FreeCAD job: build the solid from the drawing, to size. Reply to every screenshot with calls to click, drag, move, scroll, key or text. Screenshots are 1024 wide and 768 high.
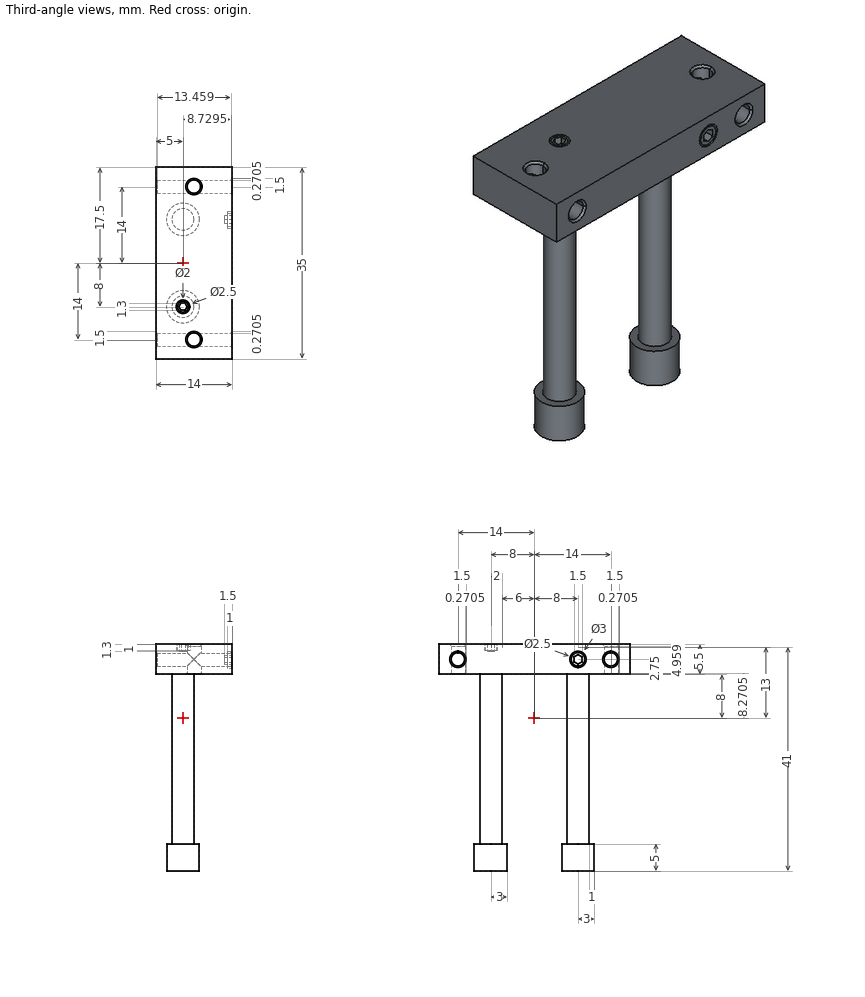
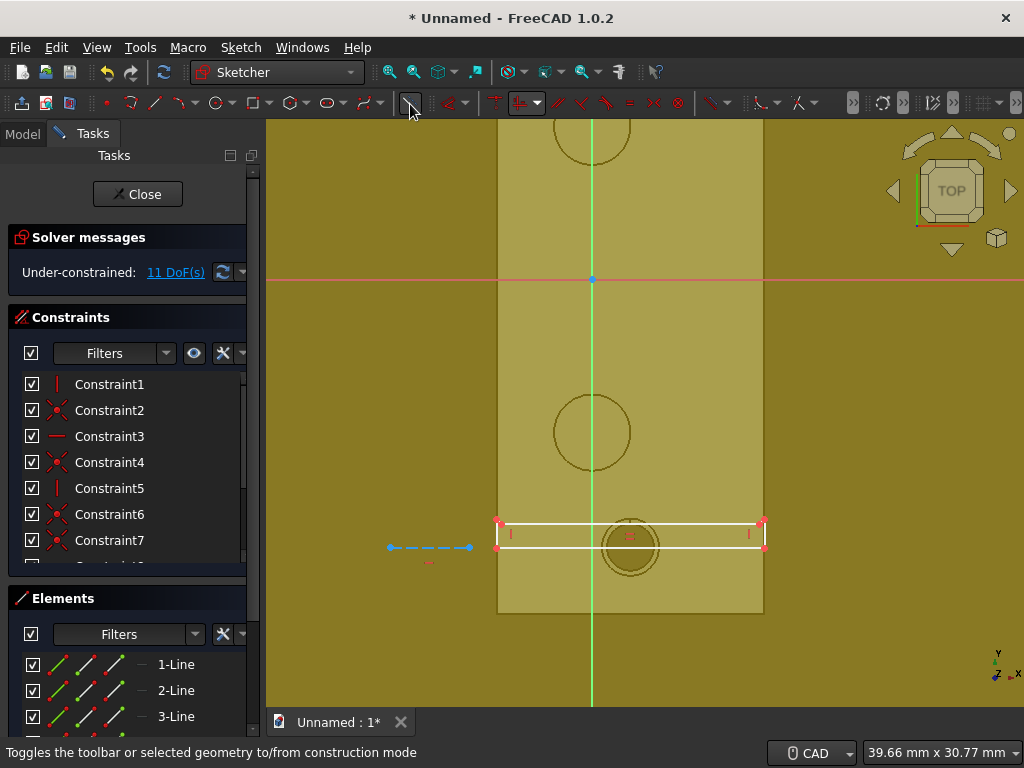
click(448, 104)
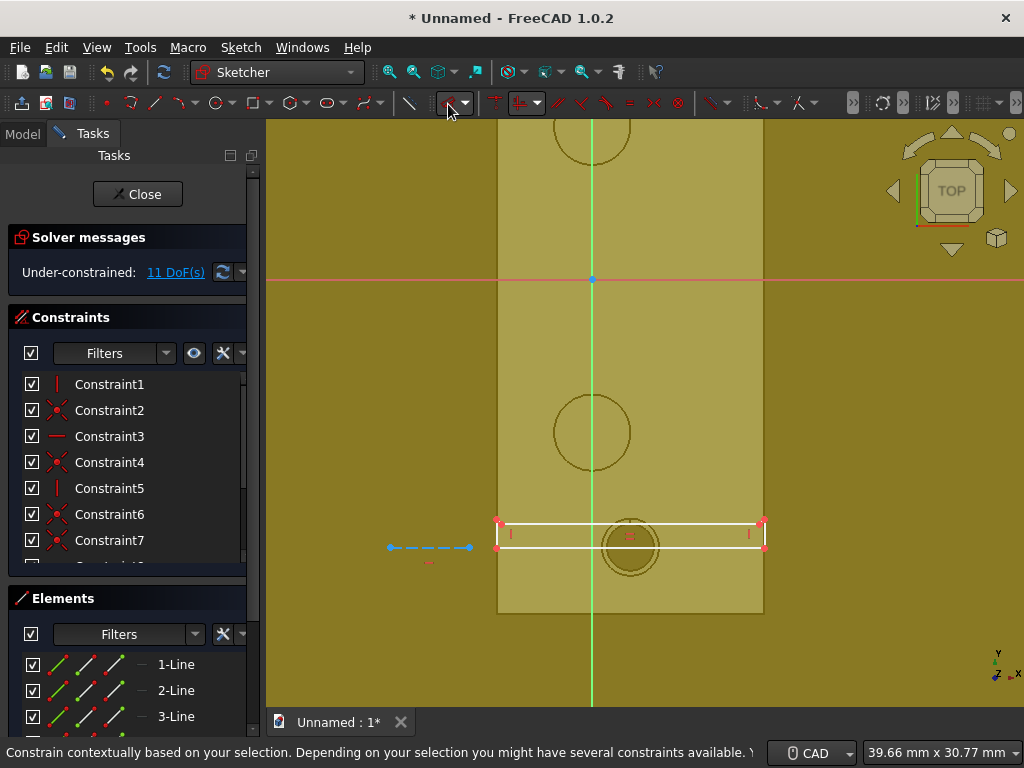
click(577, 548)
click(631, 582)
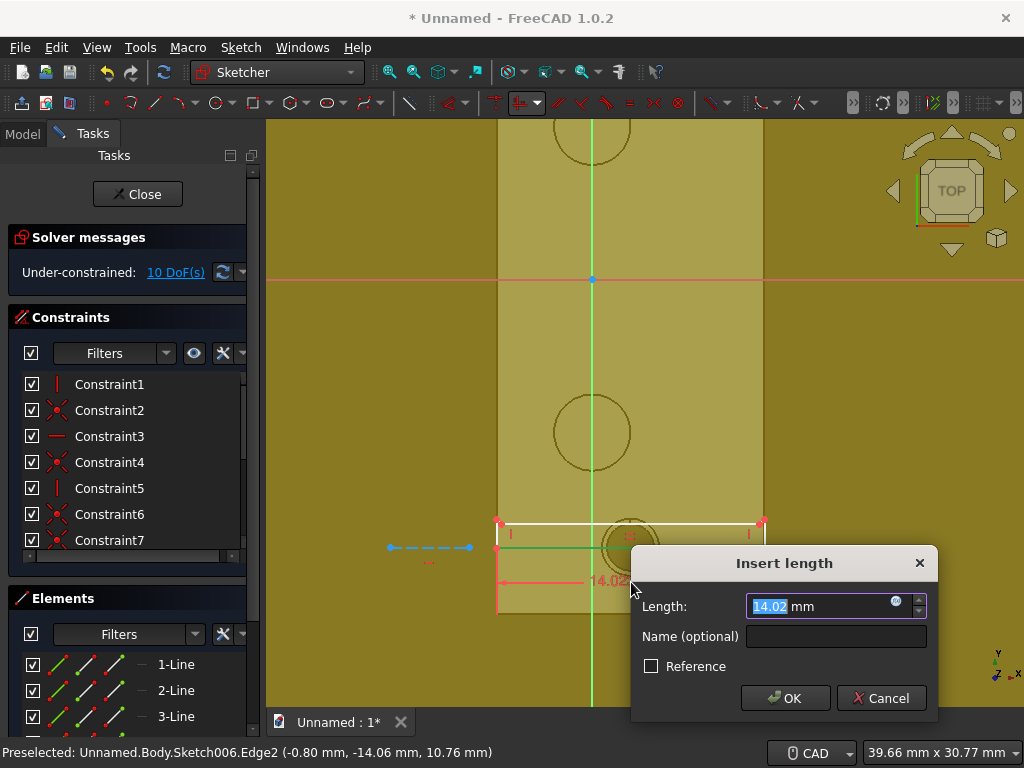
text(14)
key(Return)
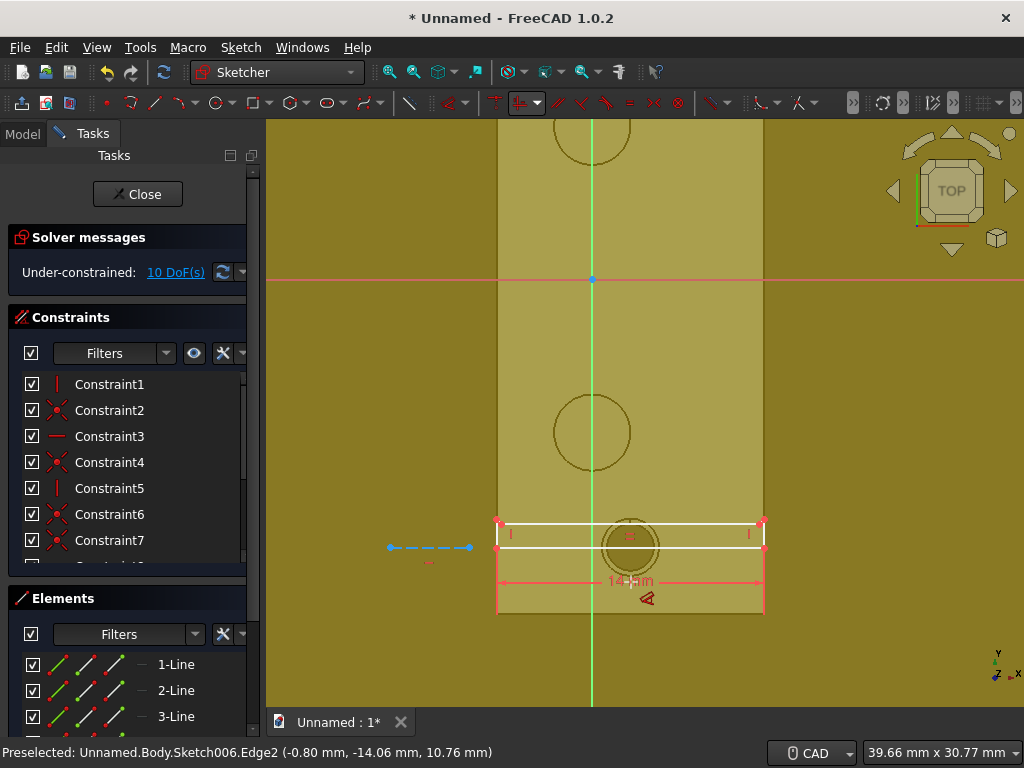
scroll(497, 519, up, 3)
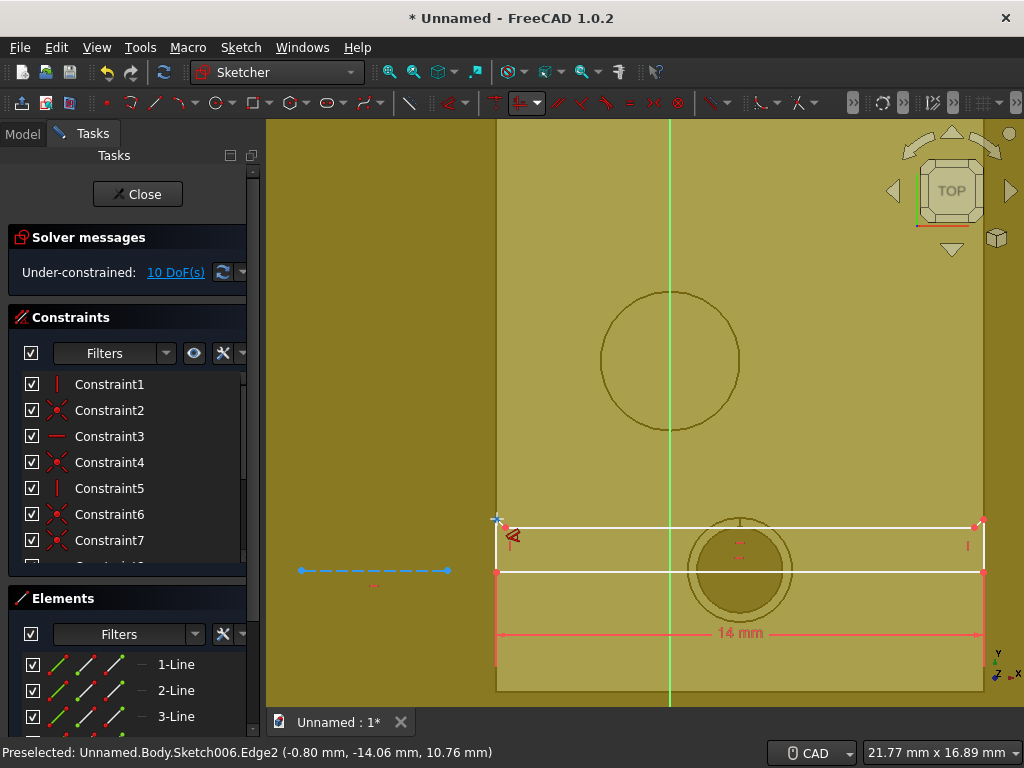
click(496, 519)
click(583, 553)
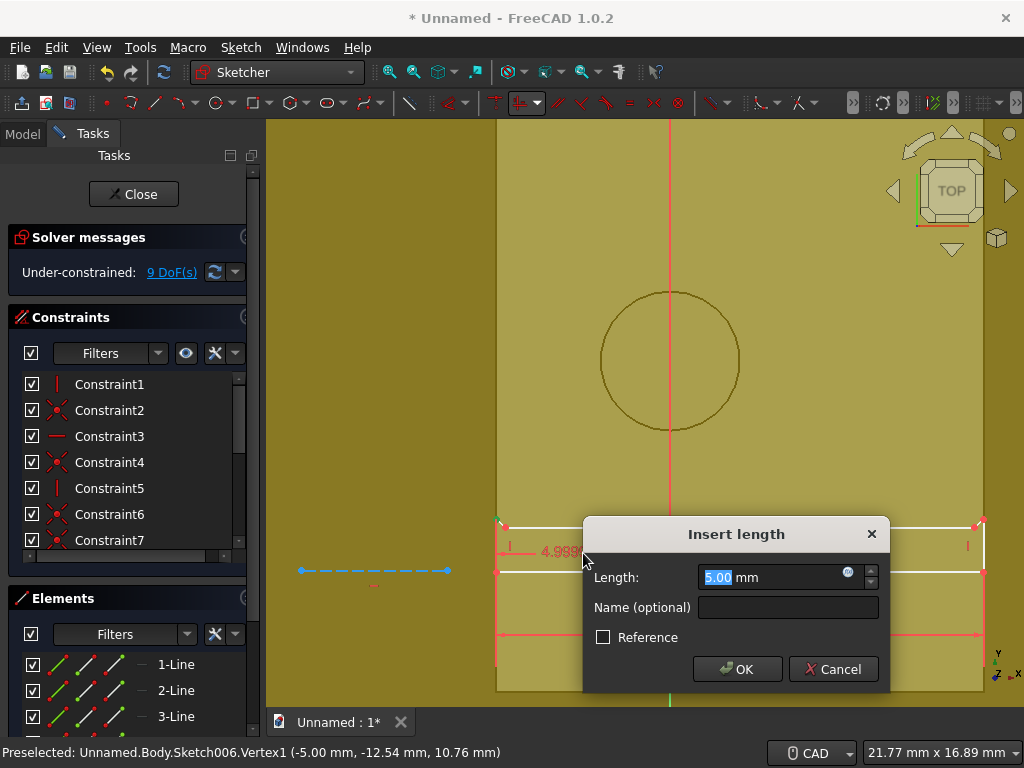
text(5)
key(Return)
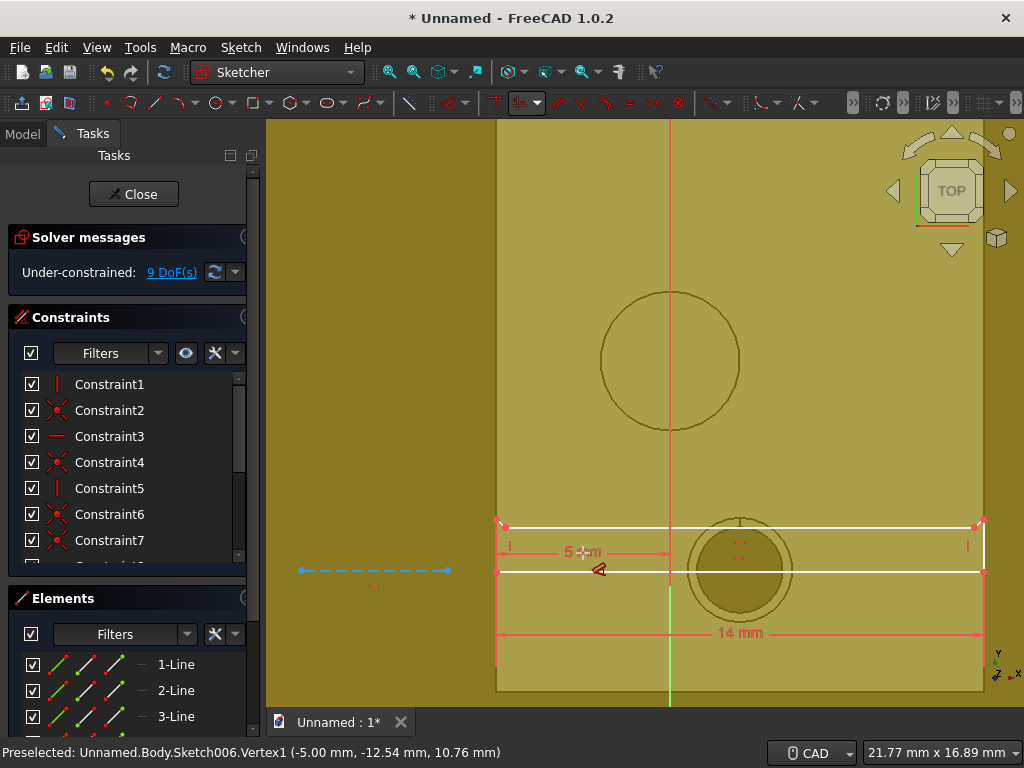
click(496, 535)
click(462, 546)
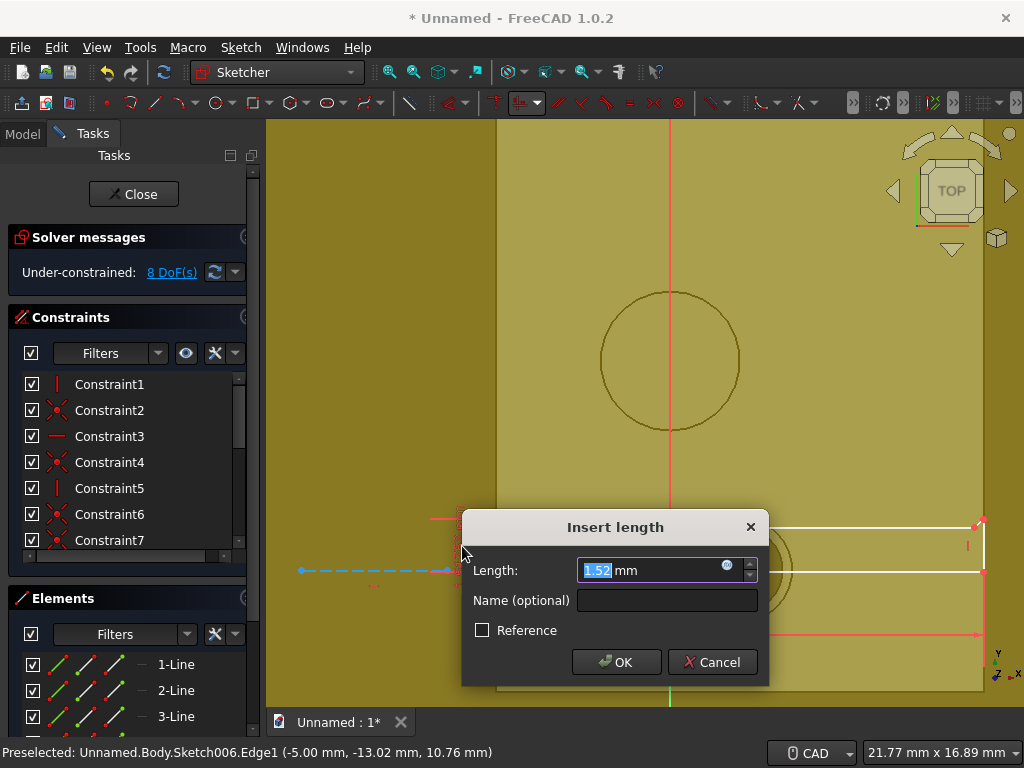
text(1.5)
key(Return)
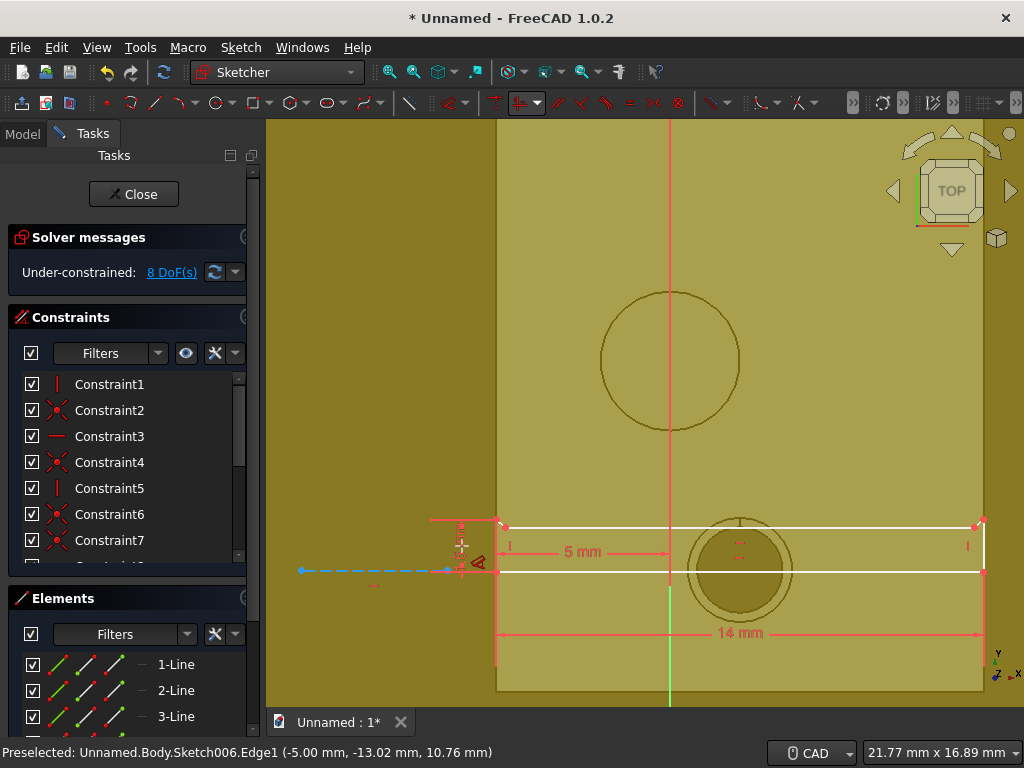
scroll(496, 519, down, 3)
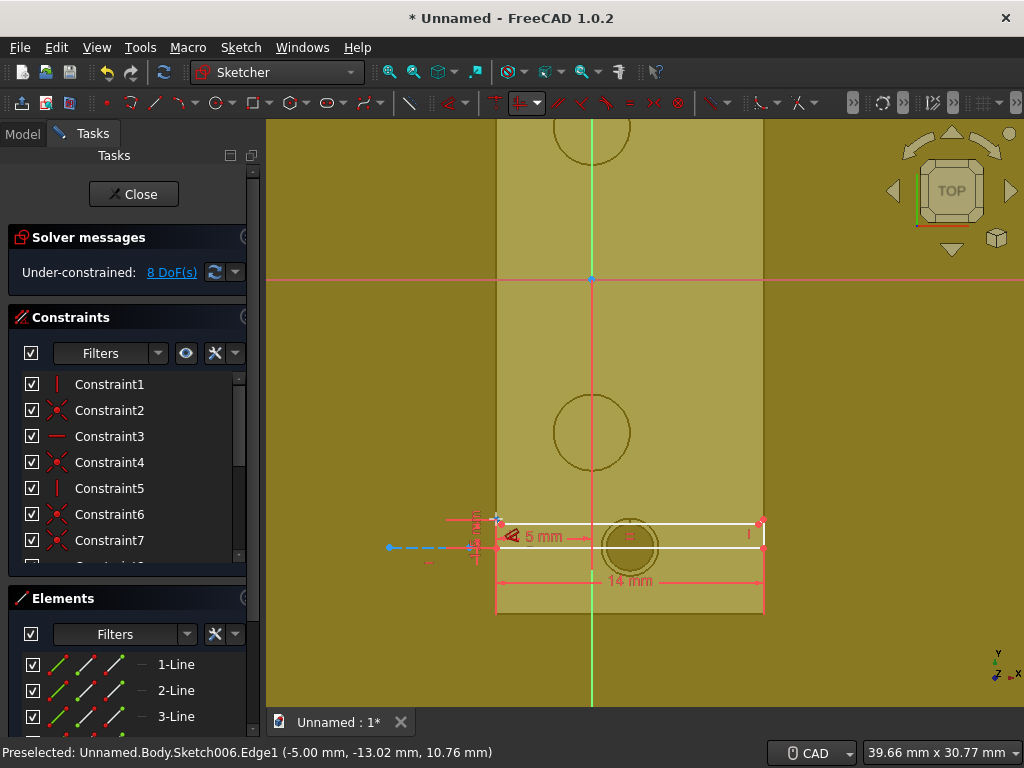
scroll(764, 540, up, 3)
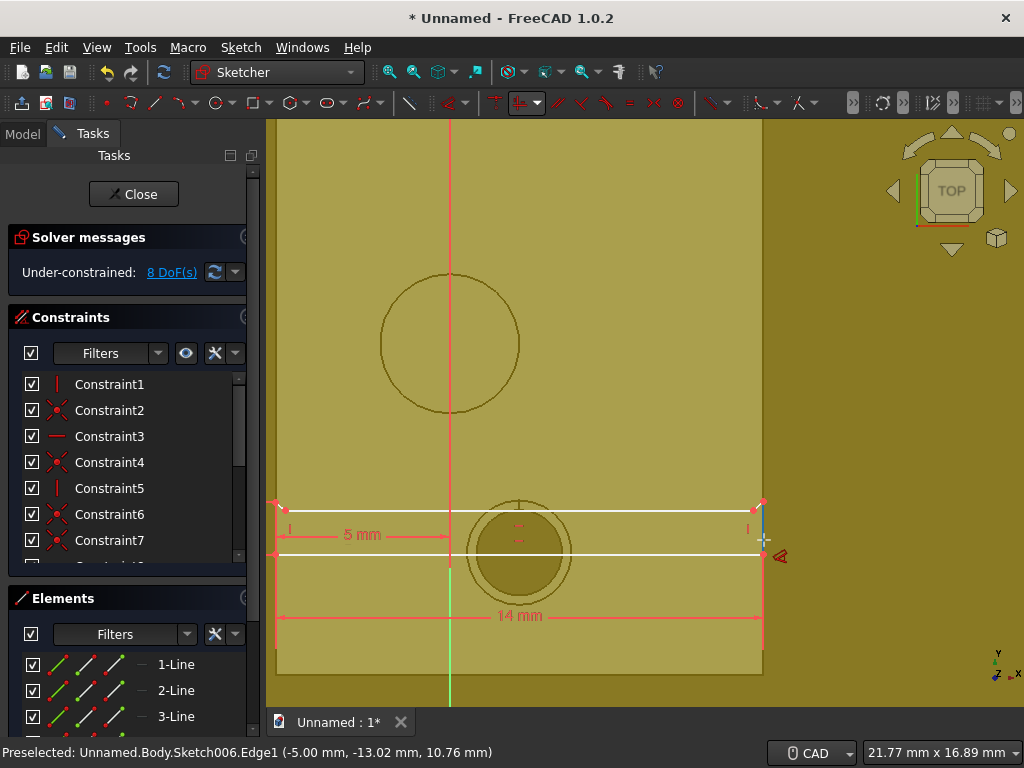
click(763, 539)
click(797, 528)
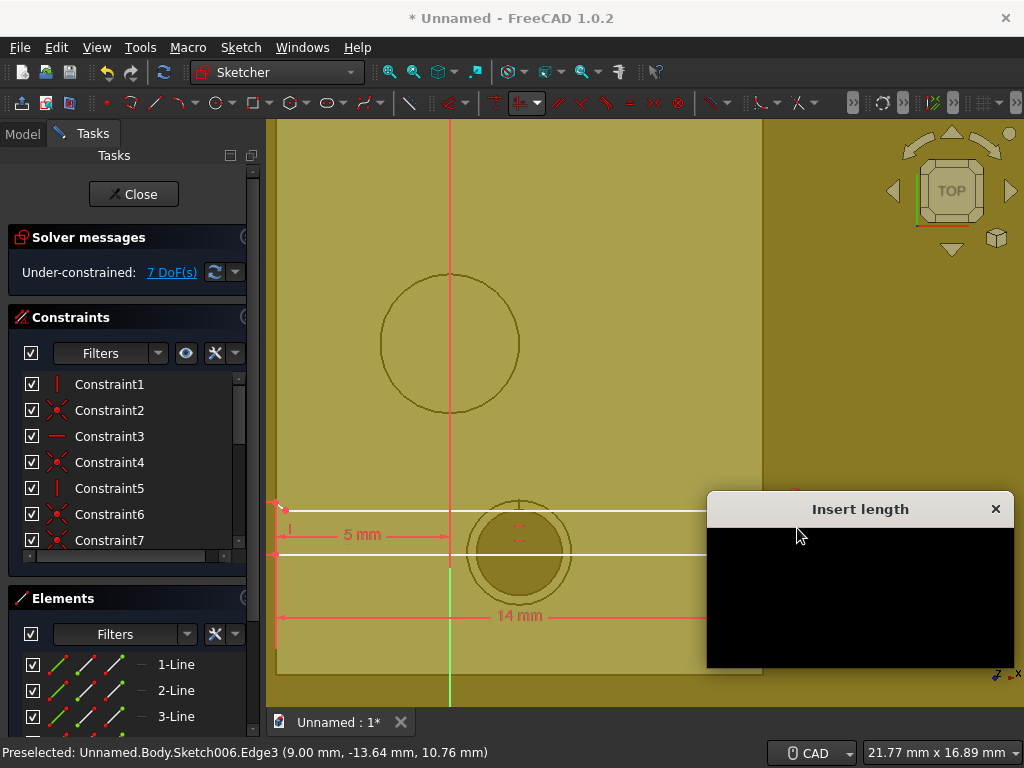
text(1.5)
key(Return)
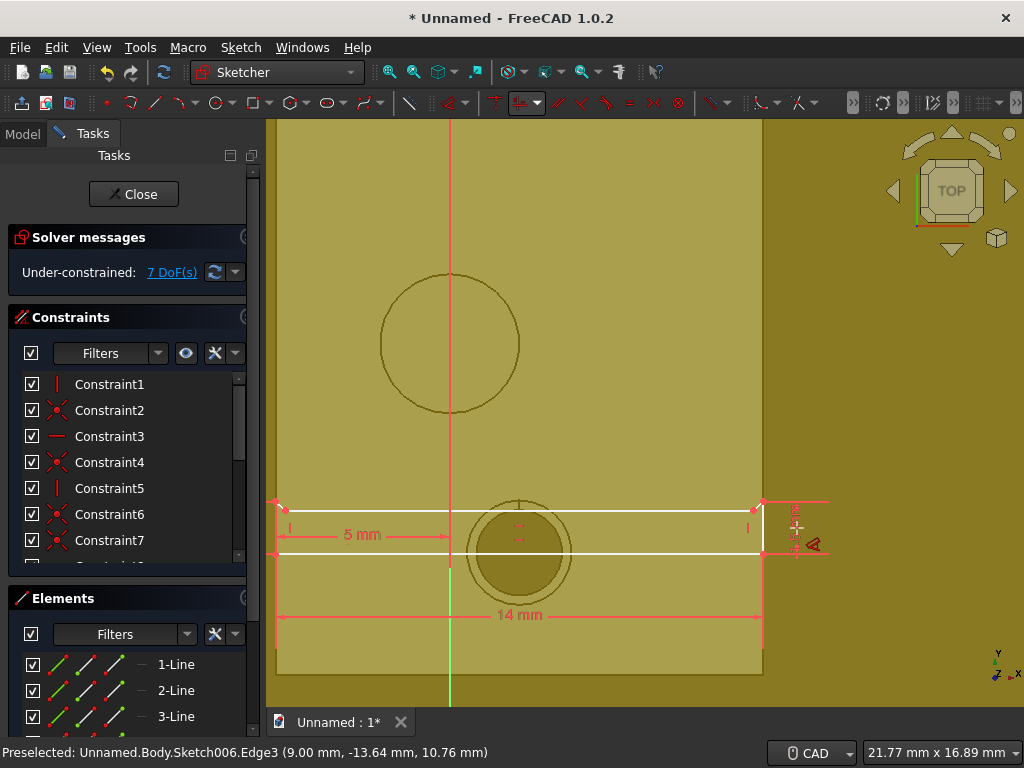
scroll(765, 540, down, 3)